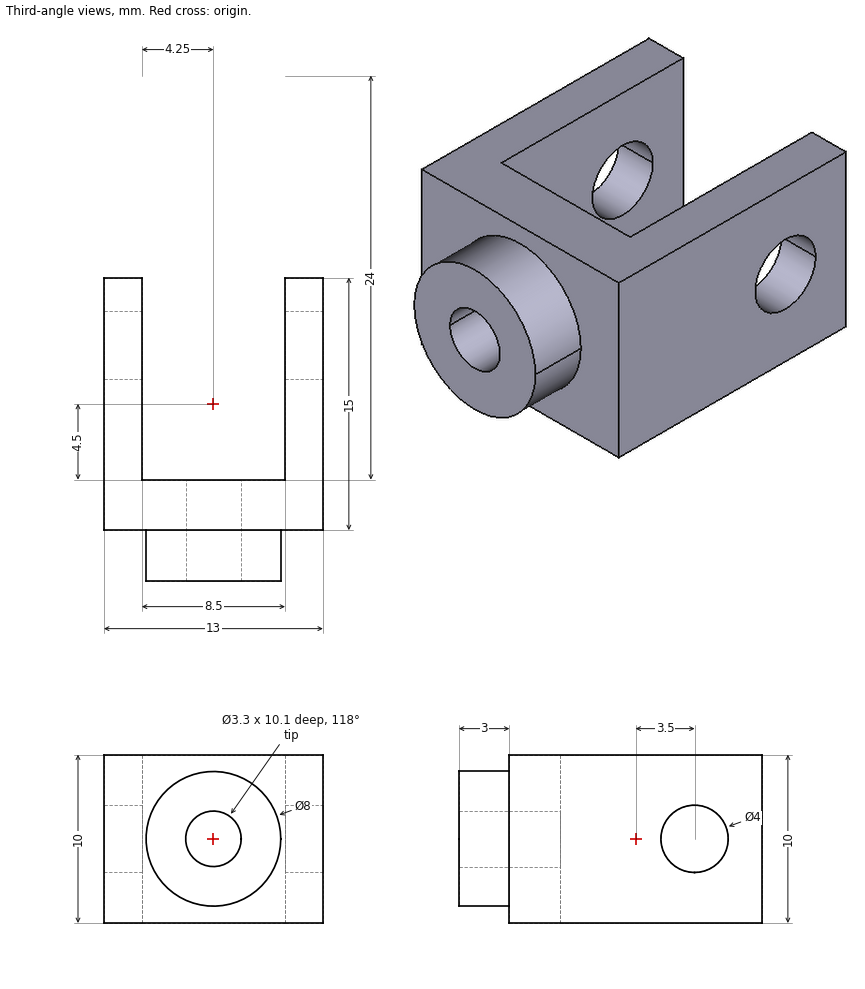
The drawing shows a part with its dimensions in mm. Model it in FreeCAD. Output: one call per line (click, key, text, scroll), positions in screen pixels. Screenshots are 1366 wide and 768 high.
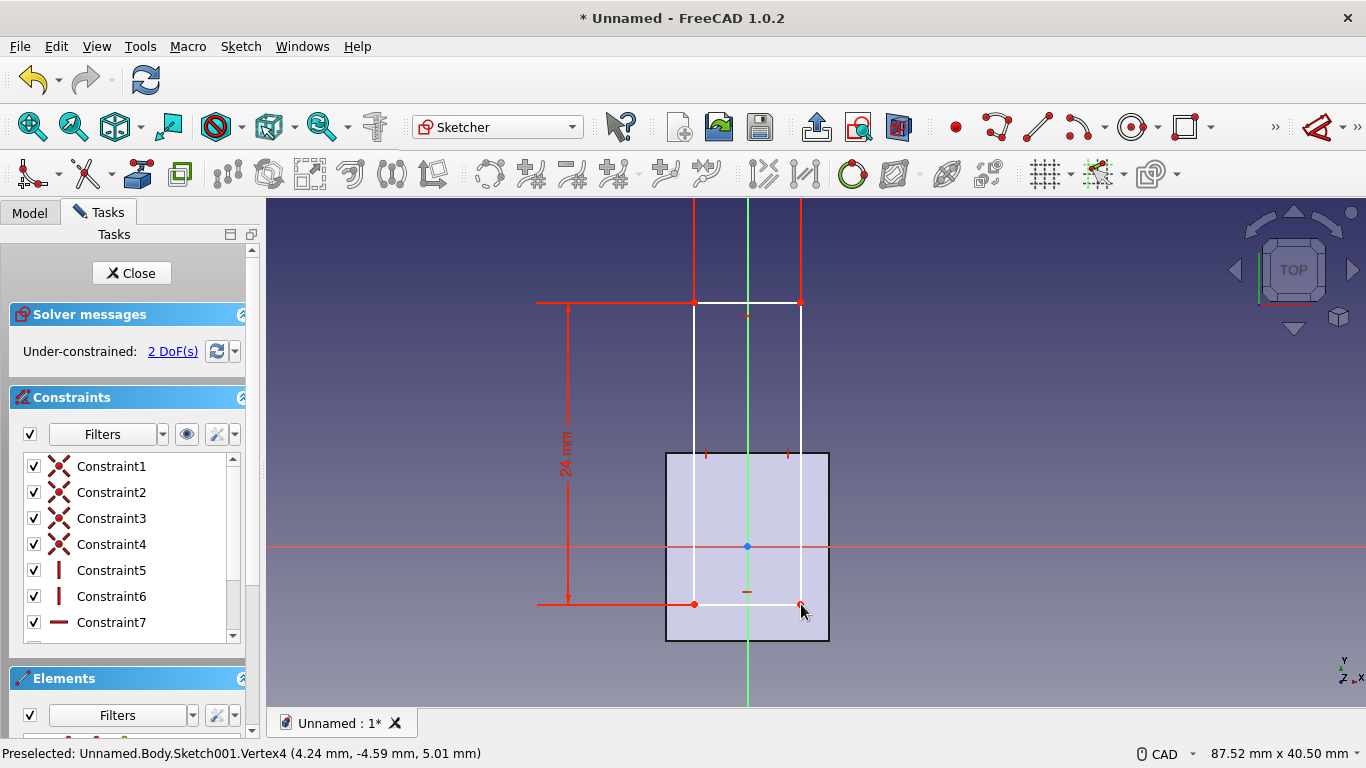
click(694, 605)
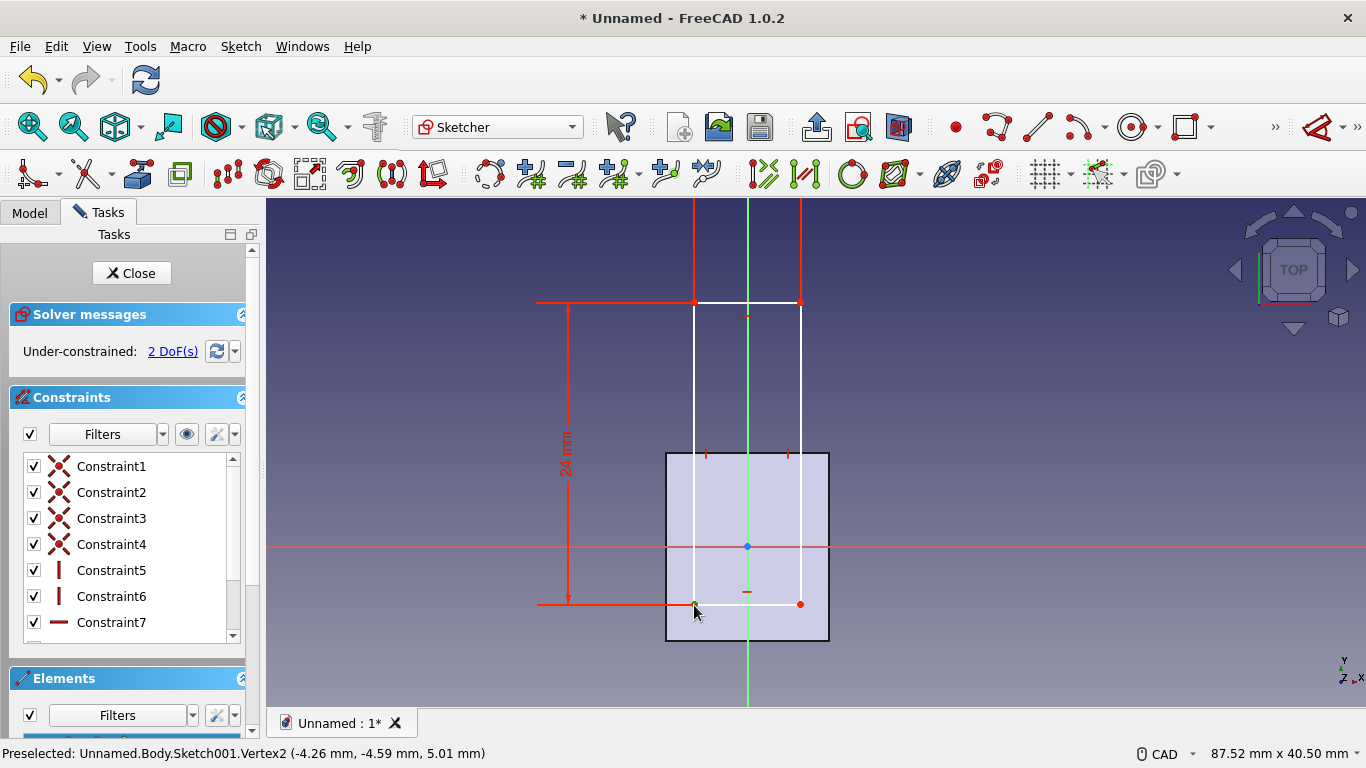
key(i)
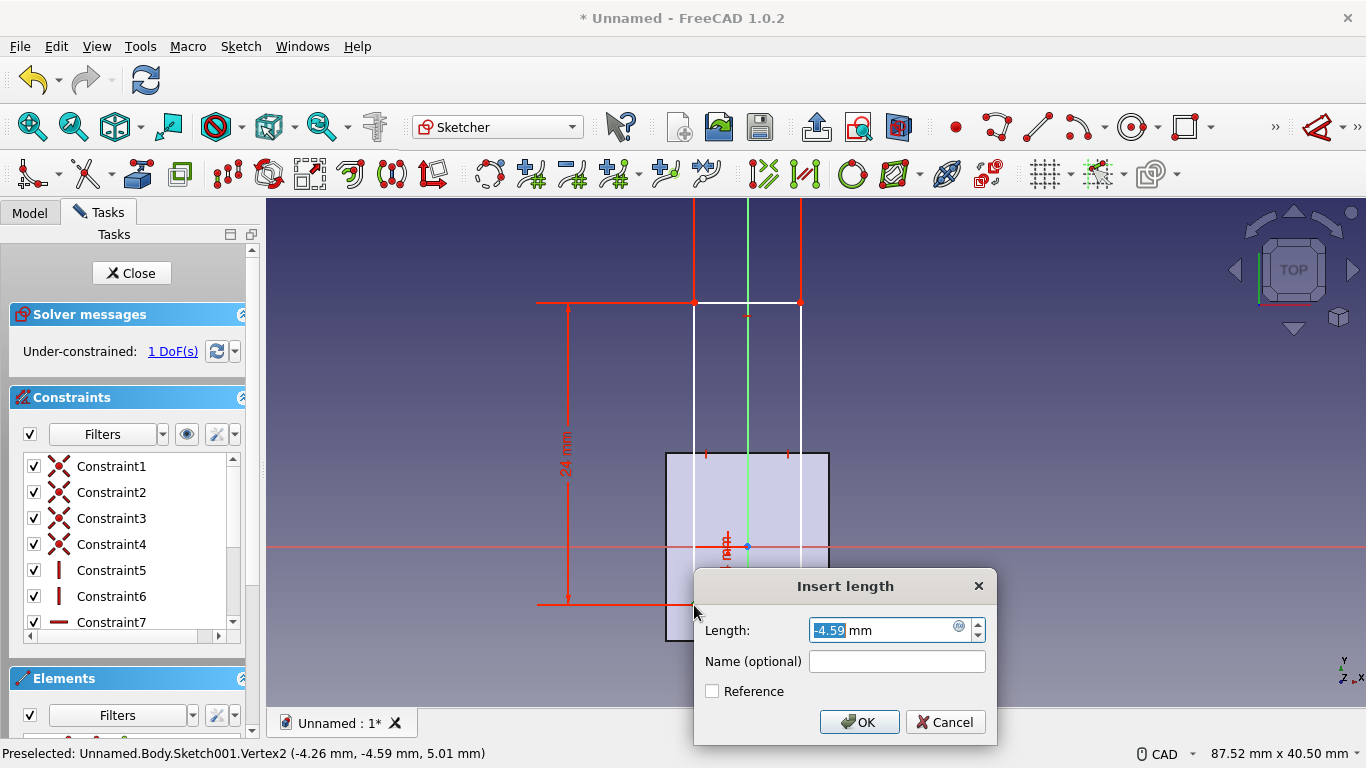
text(-4.5)
key(Return)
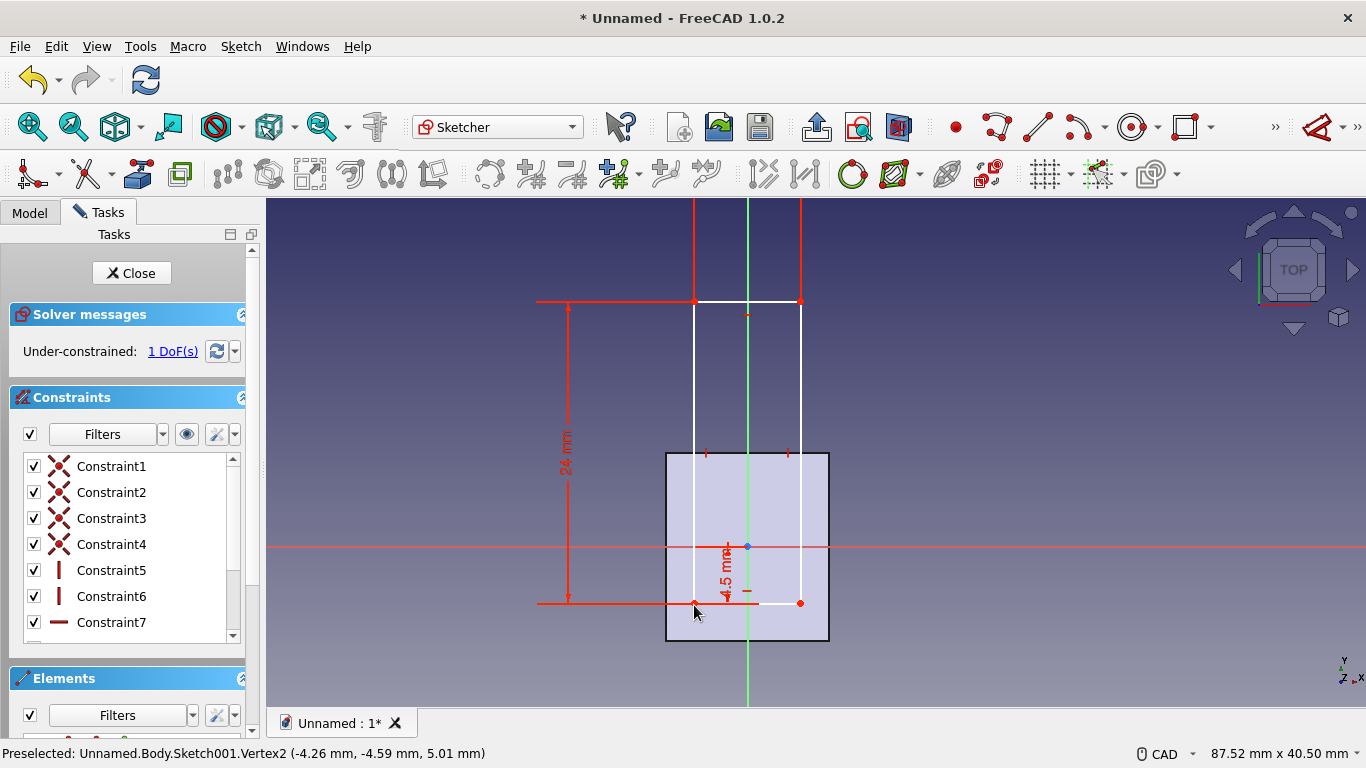
click(694, 302)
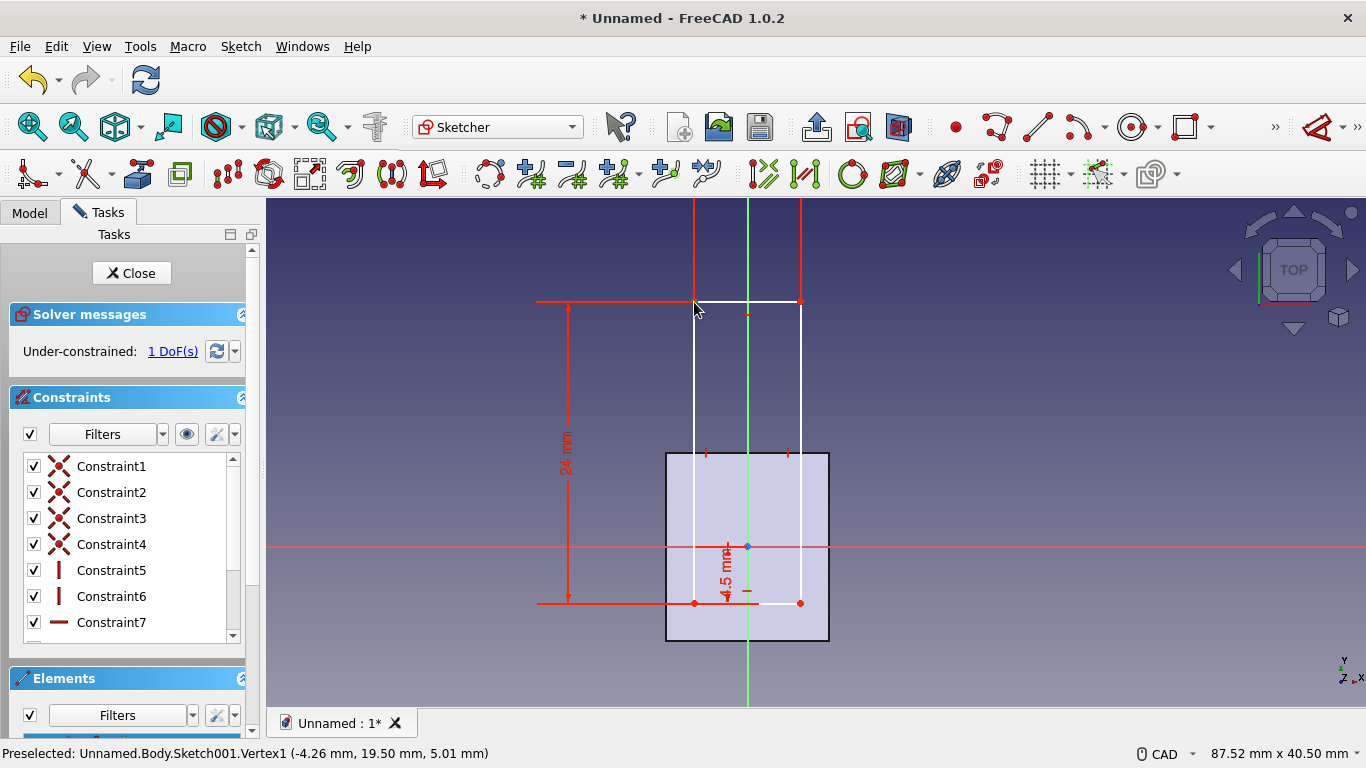
key(l)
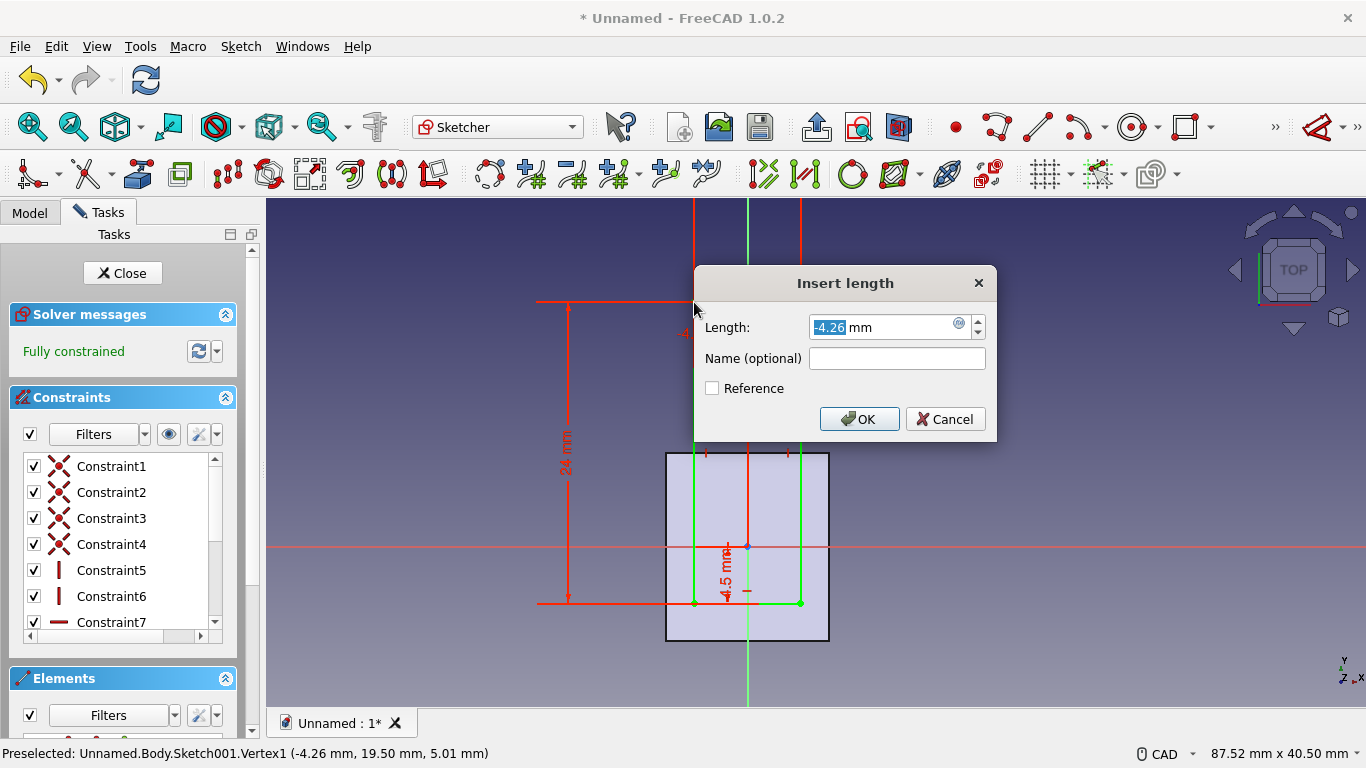
text(-4.25)
key(Return)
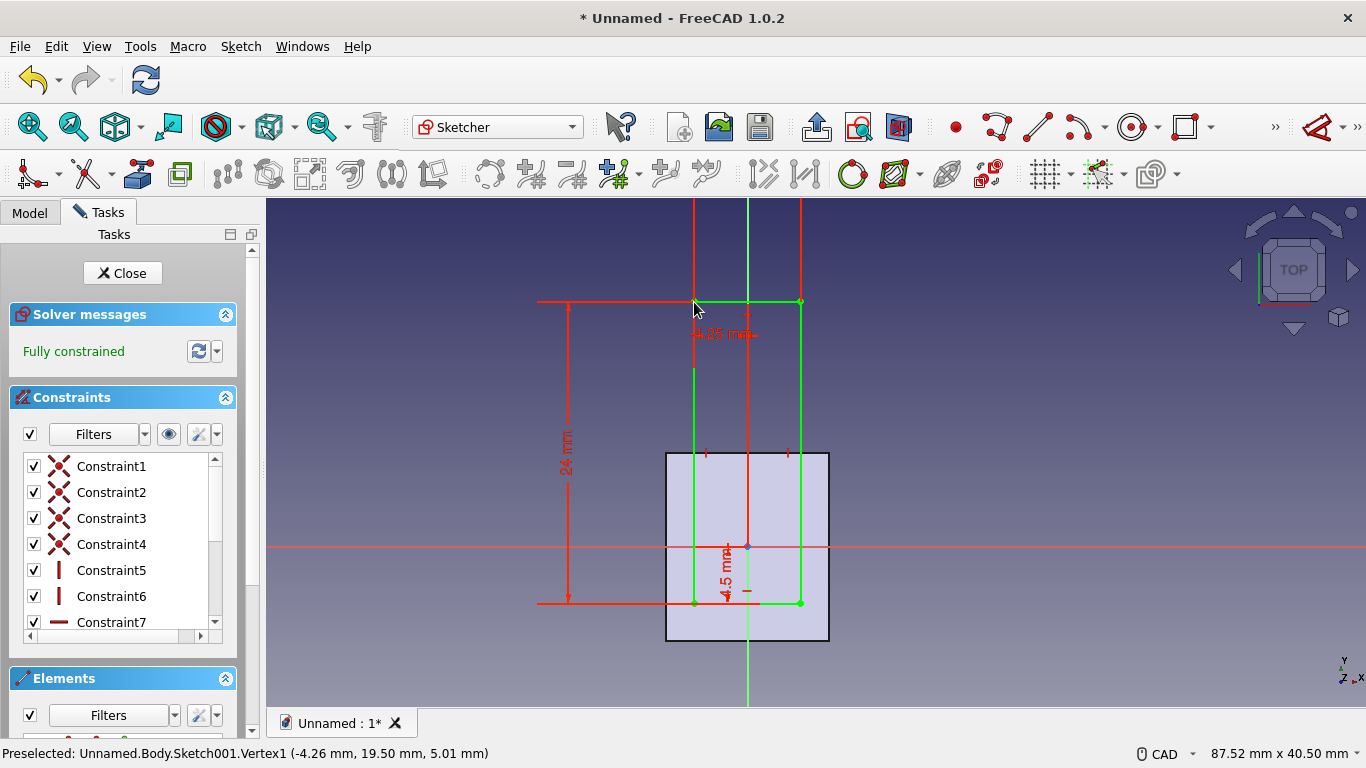
click(123, 273)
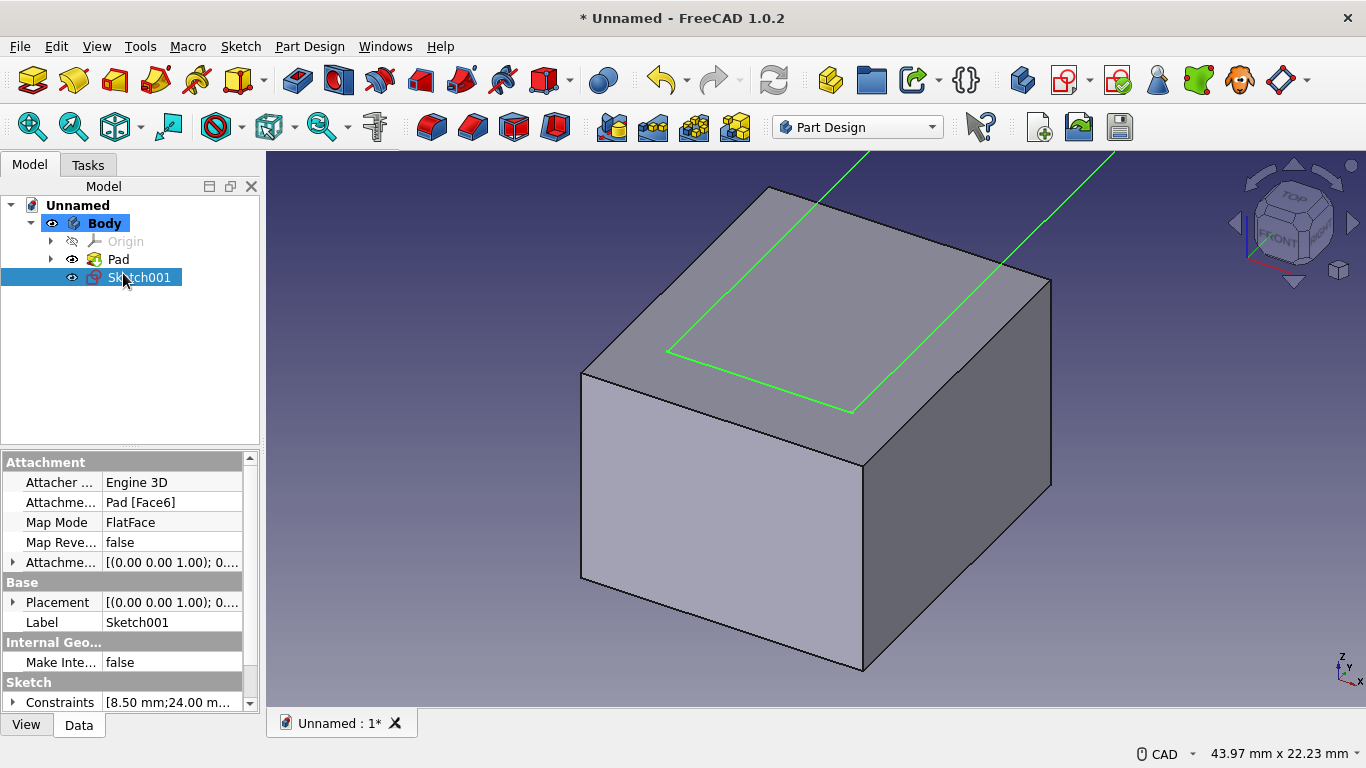
click(298, 80)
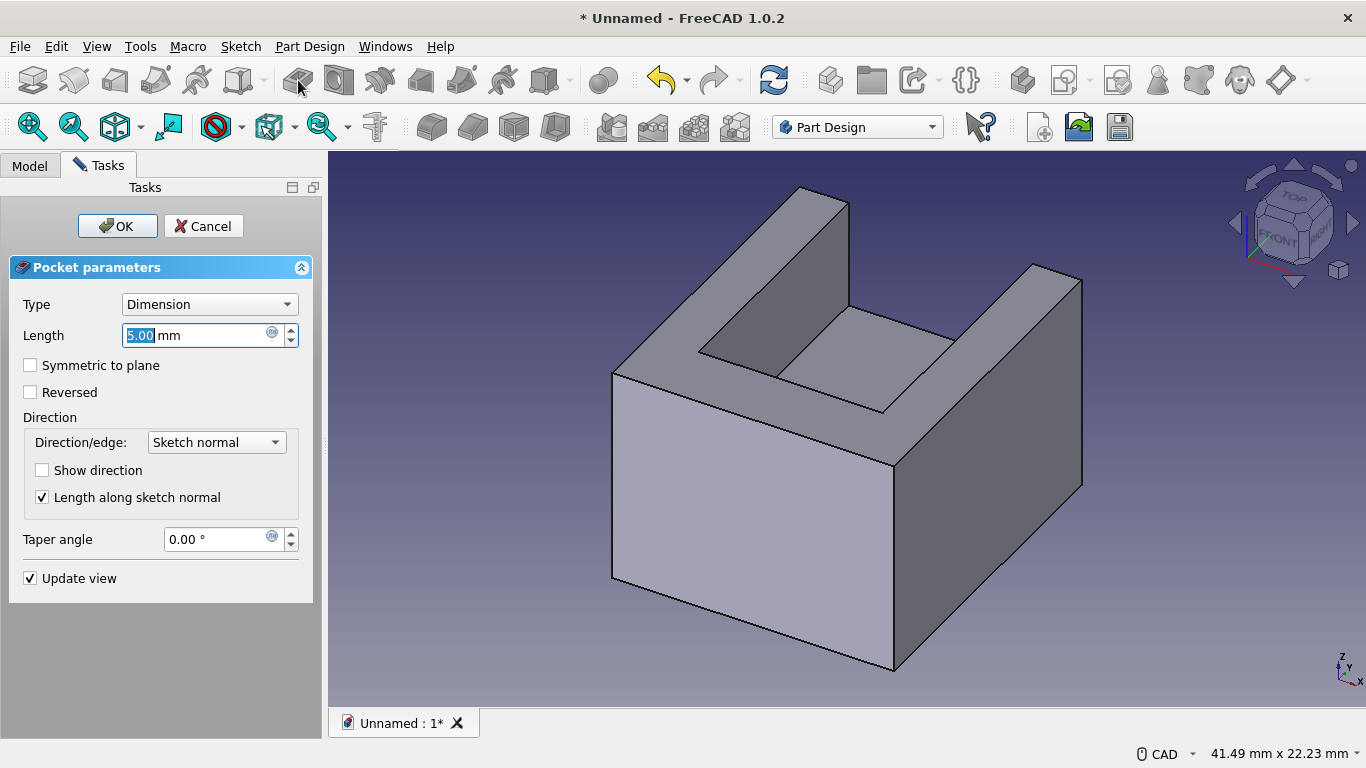
text(10)
key(Tab)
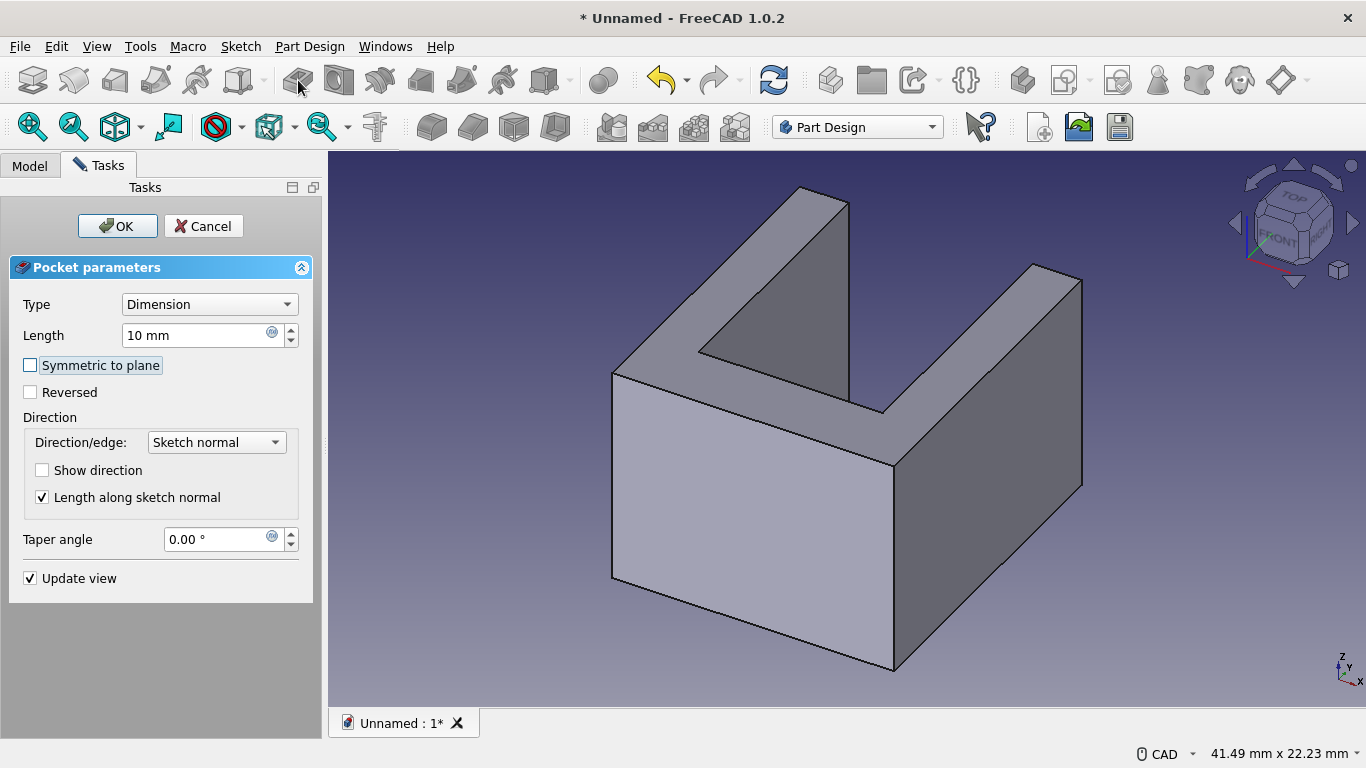
click(118, 226)